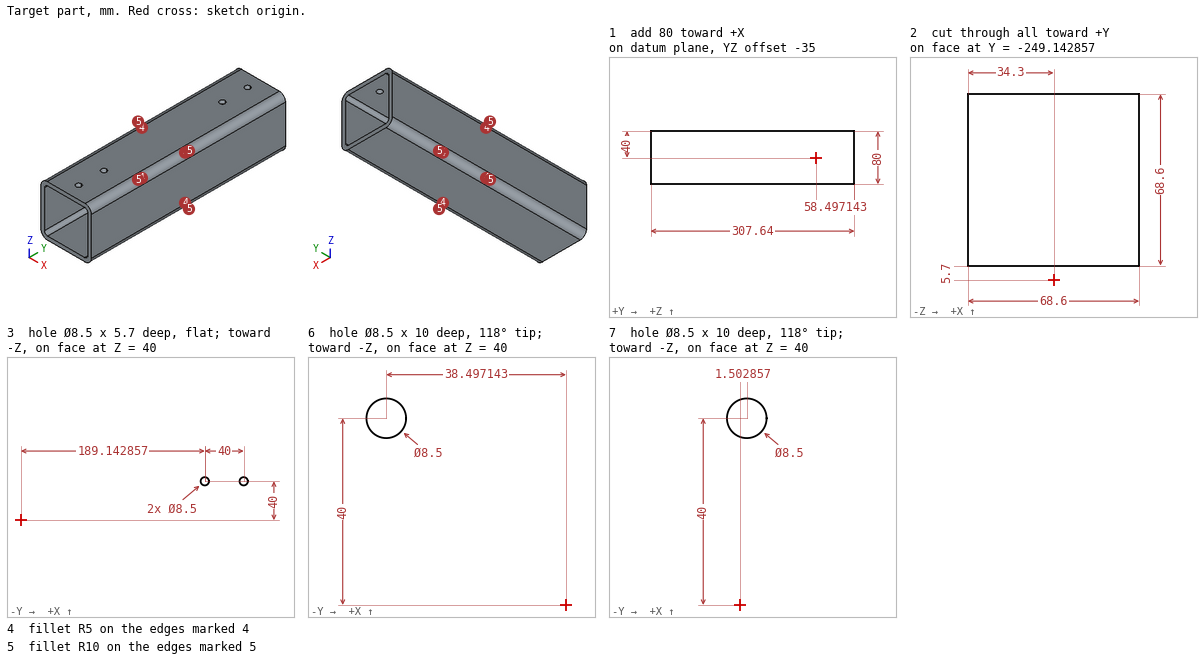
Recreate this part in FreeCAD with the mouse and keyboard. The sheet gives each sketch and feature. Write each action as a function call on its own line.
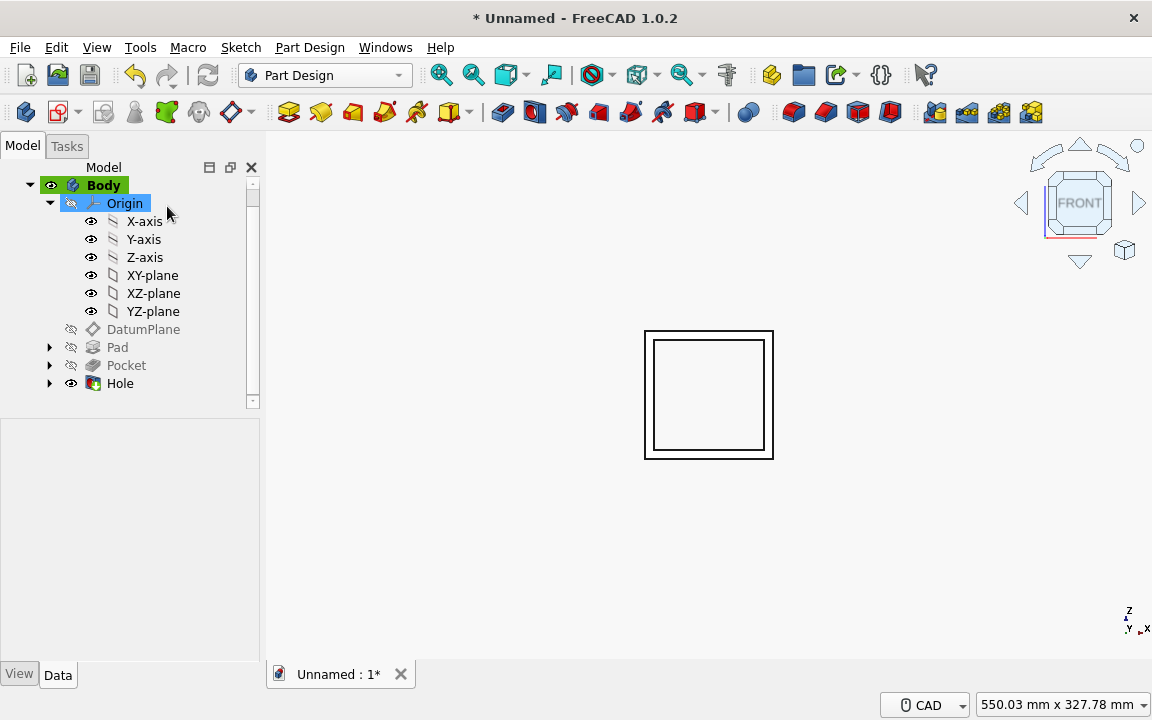
key(3)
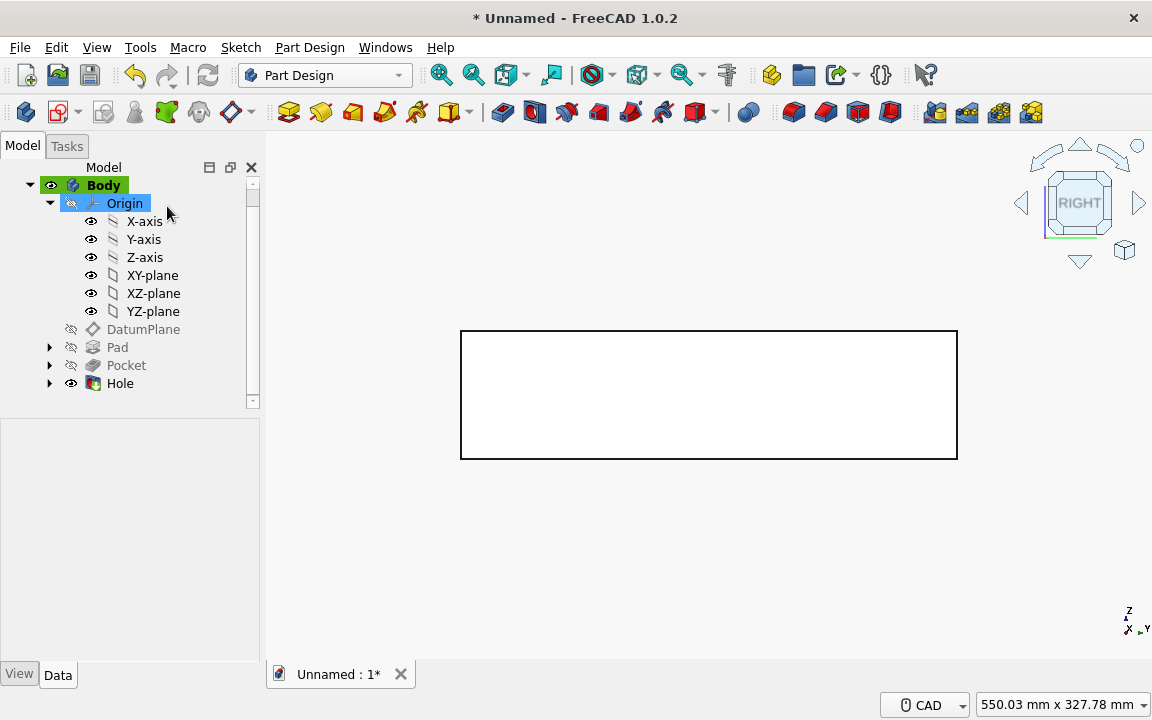
key(5)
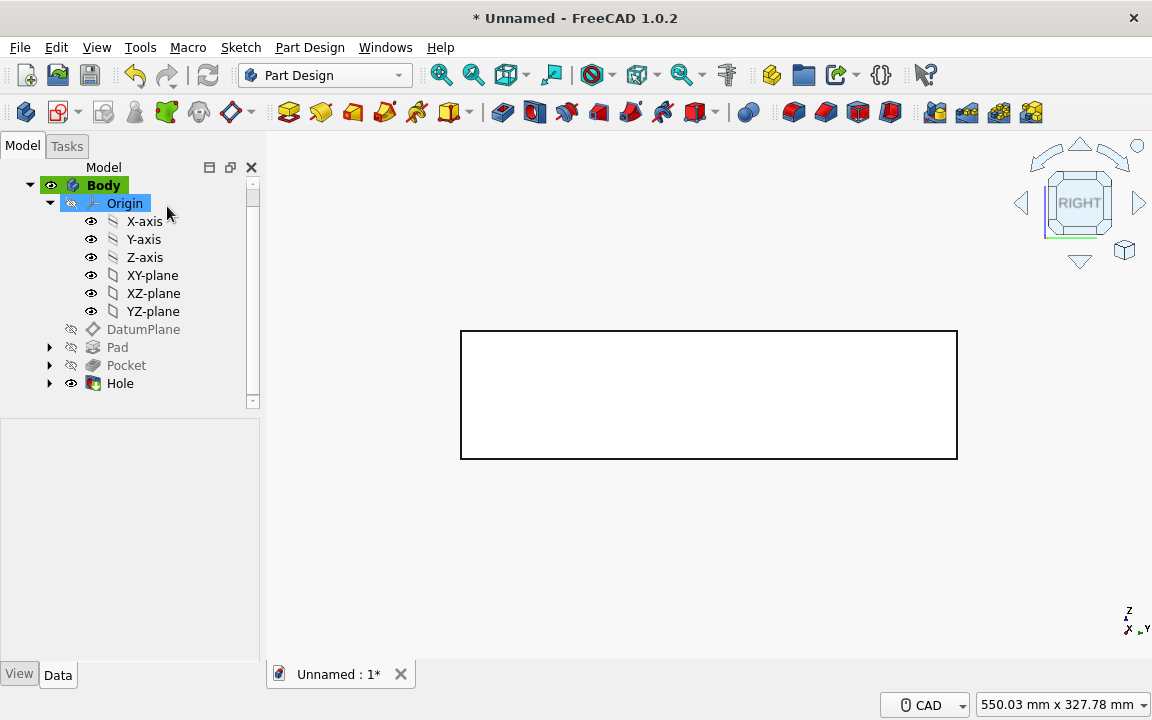
key(4)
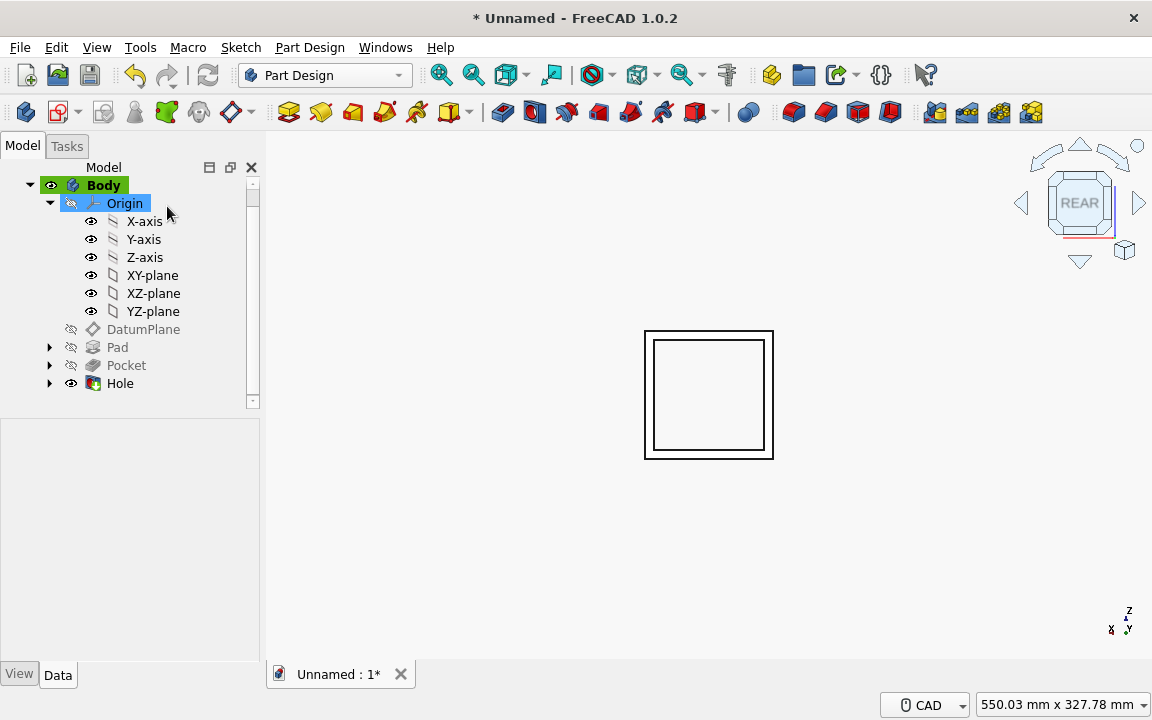
key(v)
key(f)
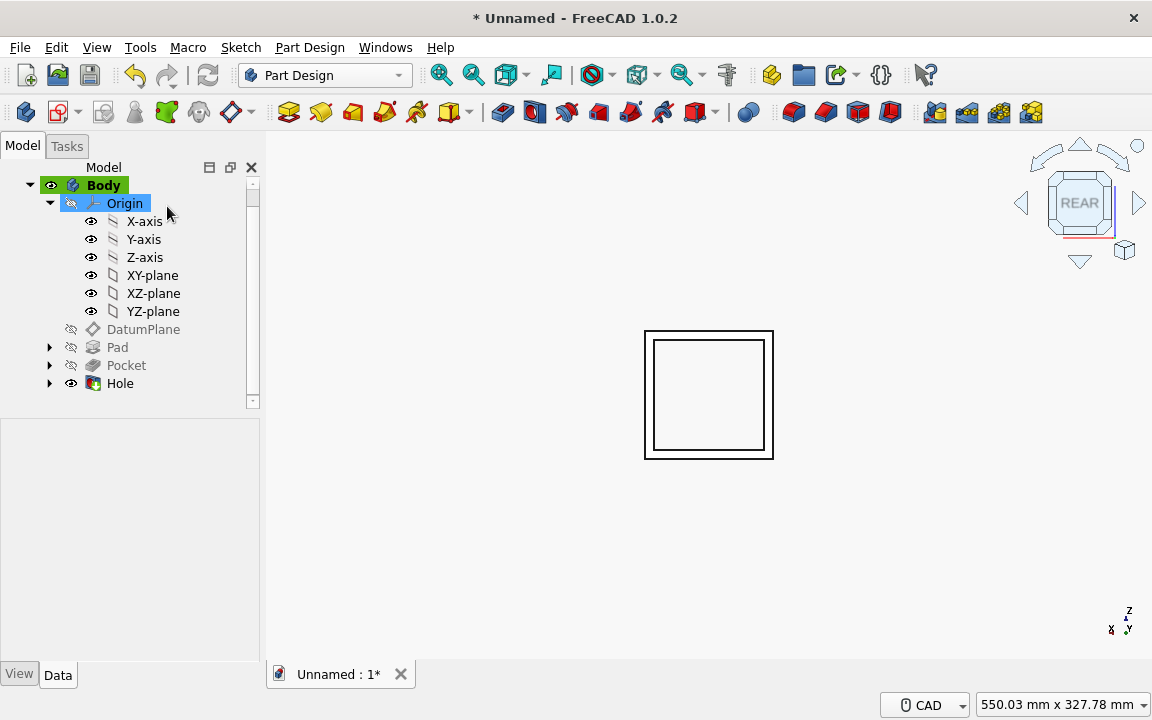
key(6)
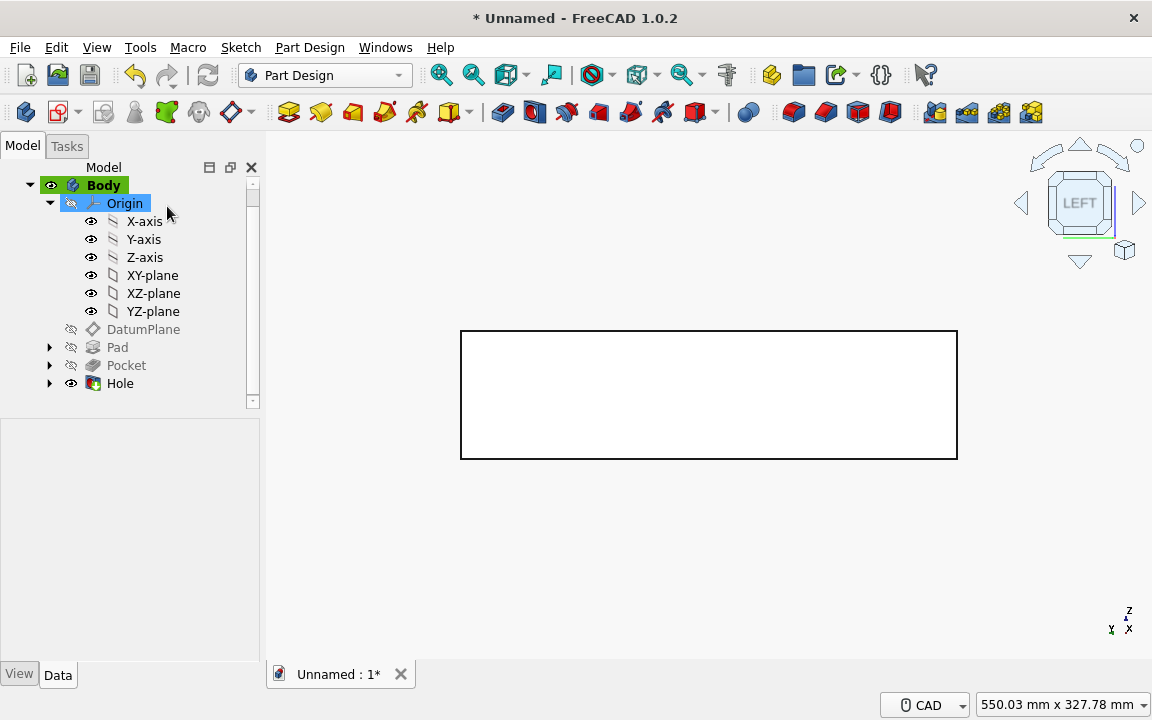
key(v)
key(3)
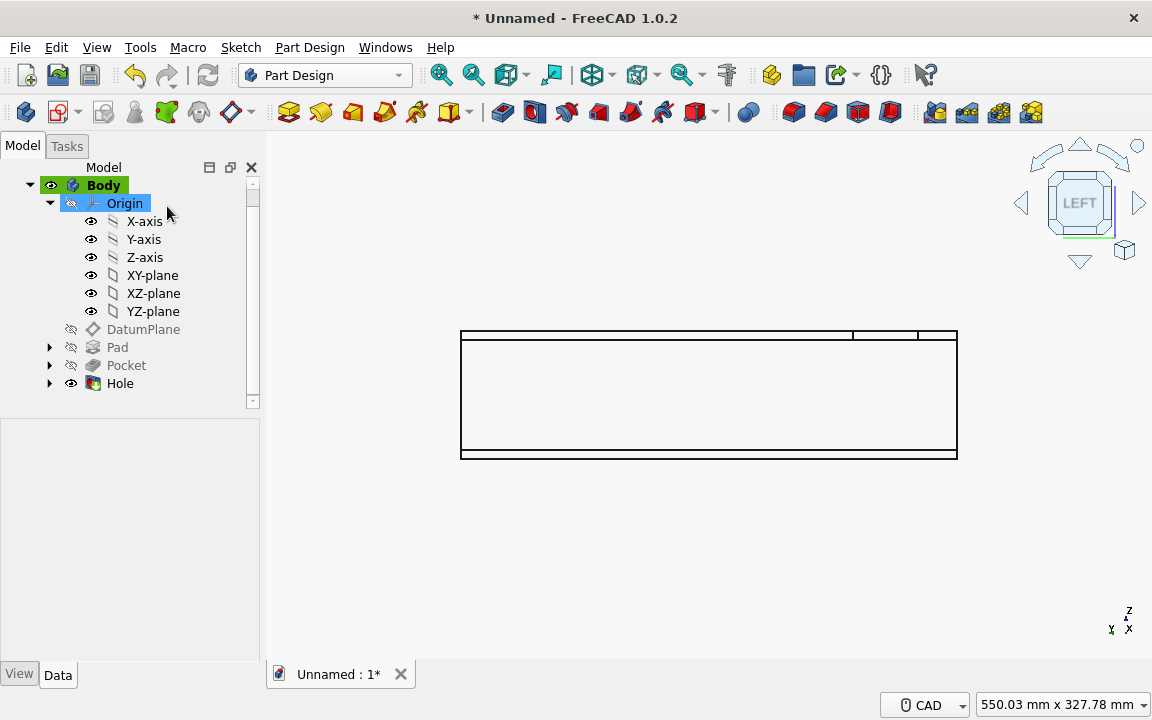
key(0)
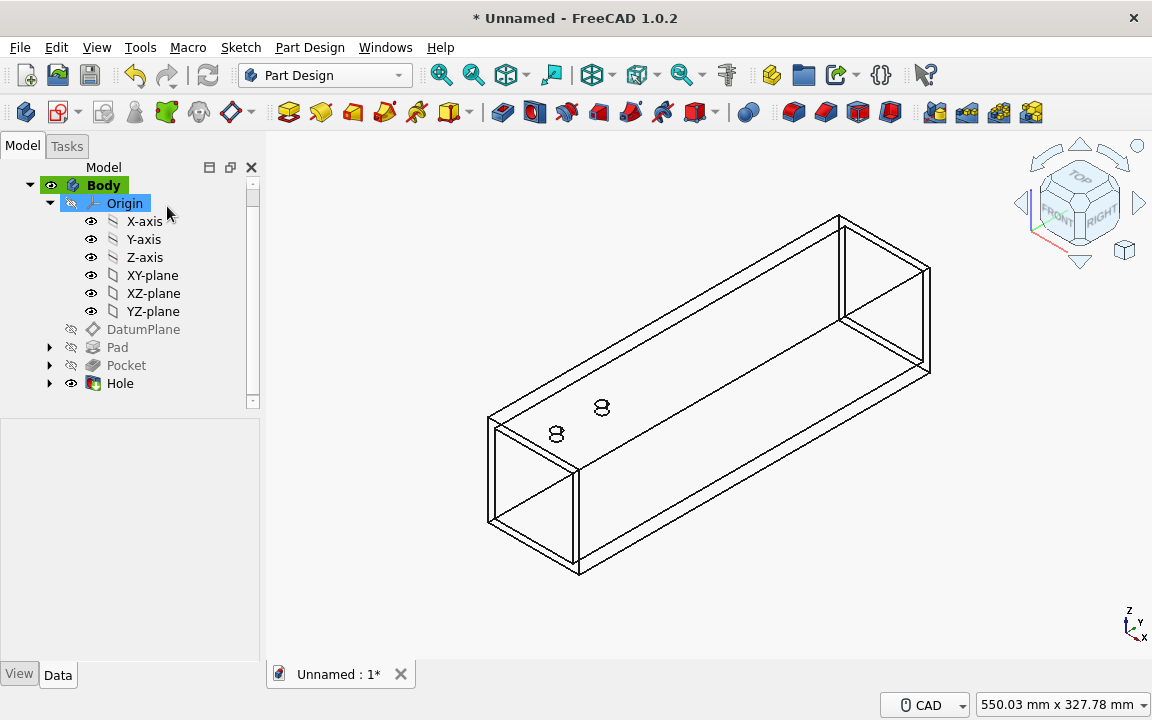
click(565, 477)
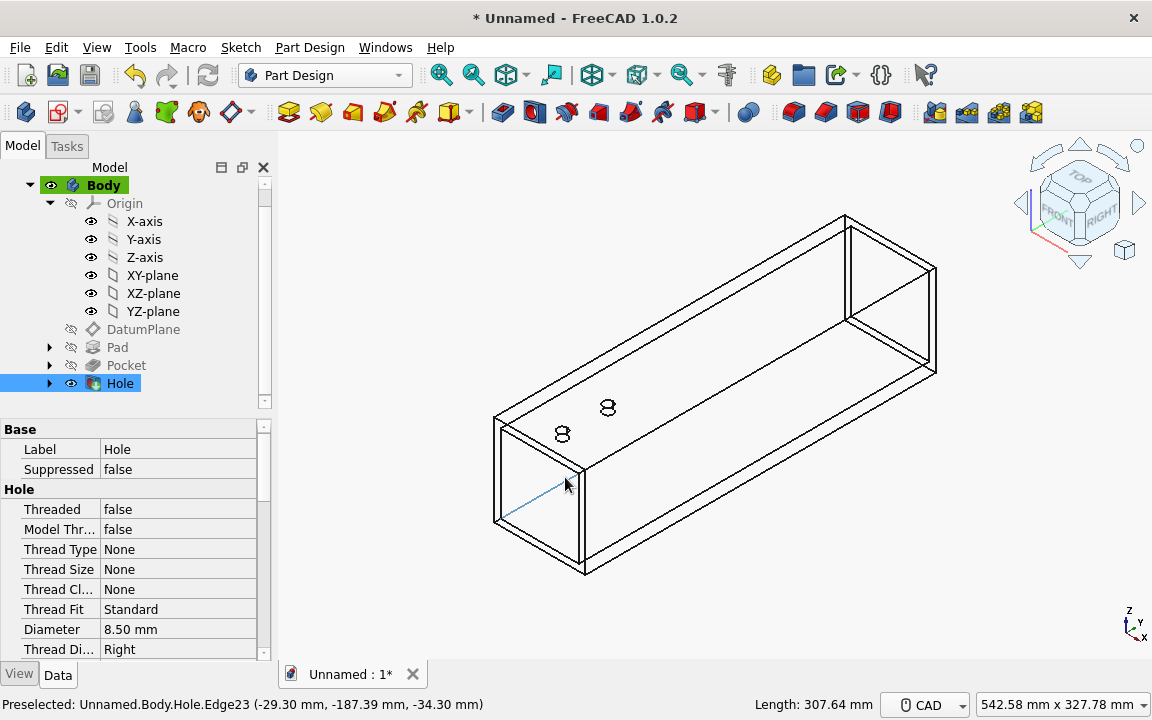
click(676, 326, ctrl)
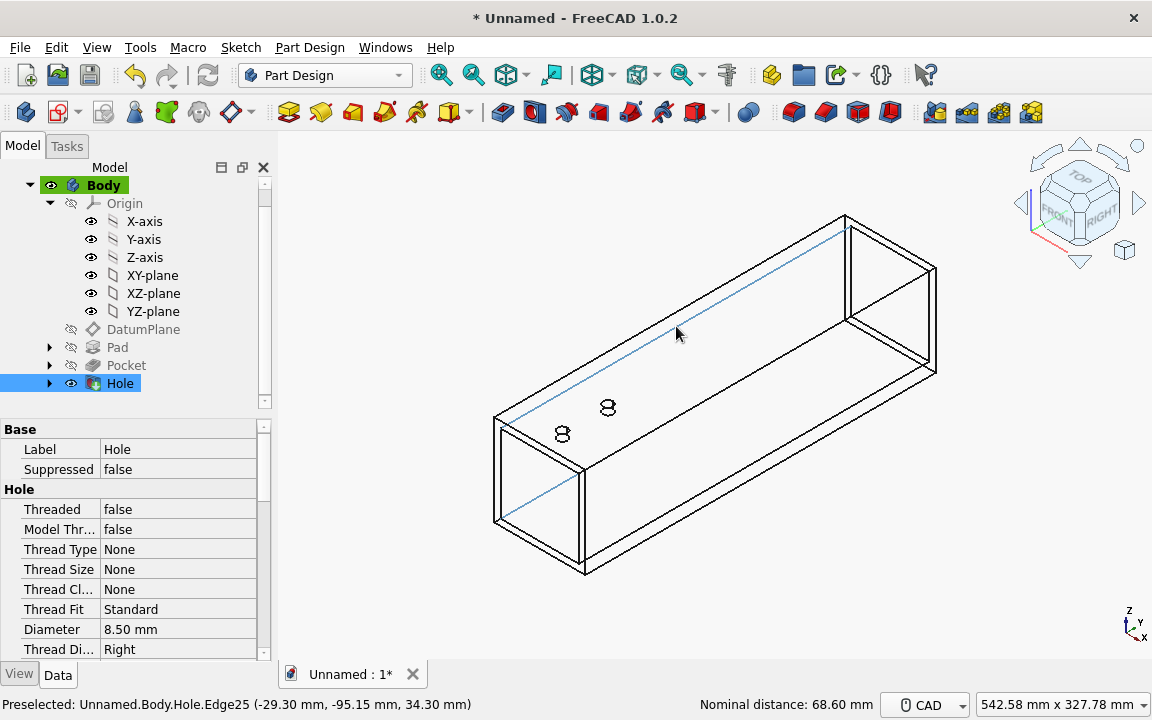
click(754, 462, ctrl)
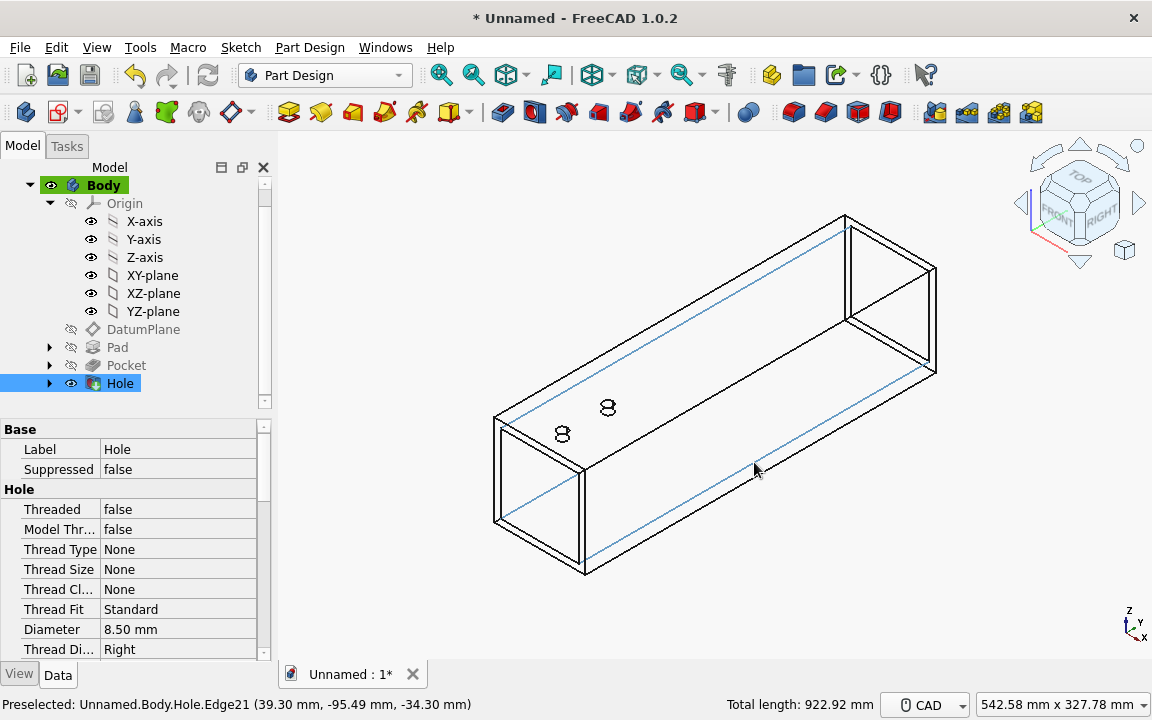
key(2)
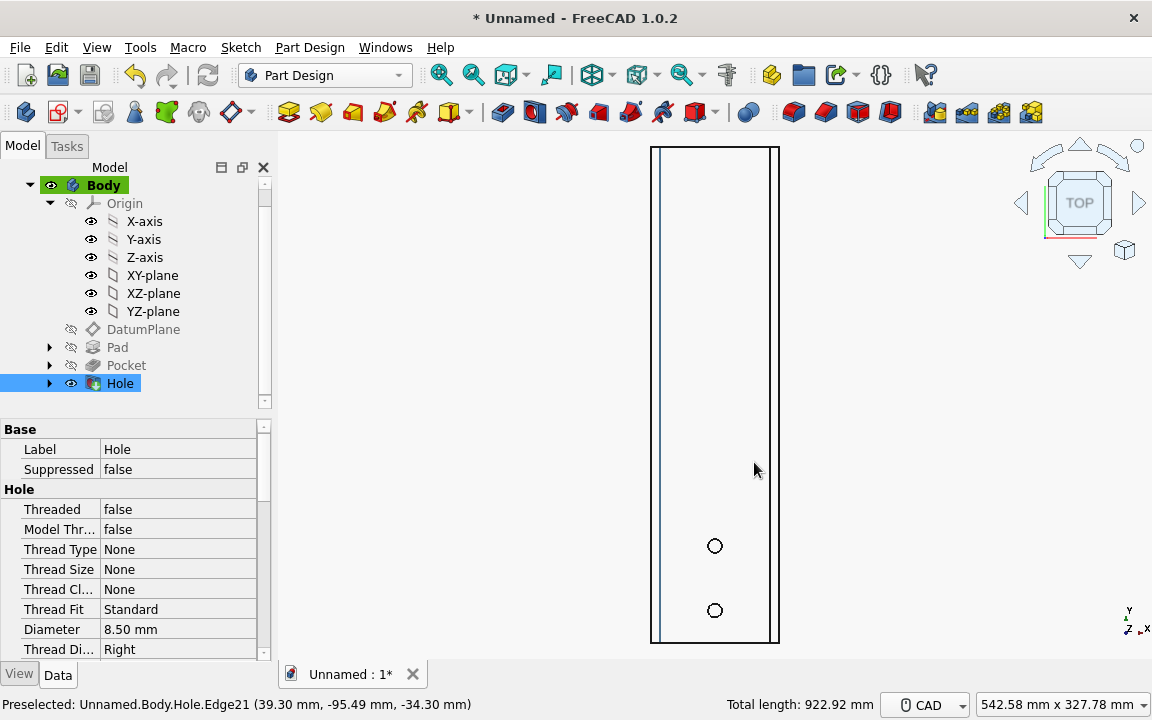
click(770, 394, ctrl)